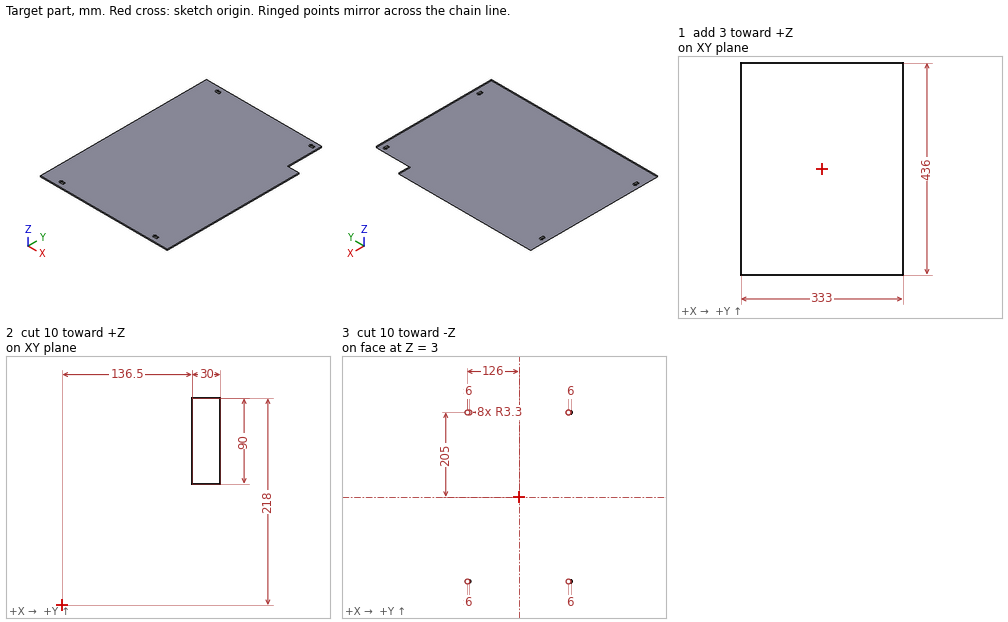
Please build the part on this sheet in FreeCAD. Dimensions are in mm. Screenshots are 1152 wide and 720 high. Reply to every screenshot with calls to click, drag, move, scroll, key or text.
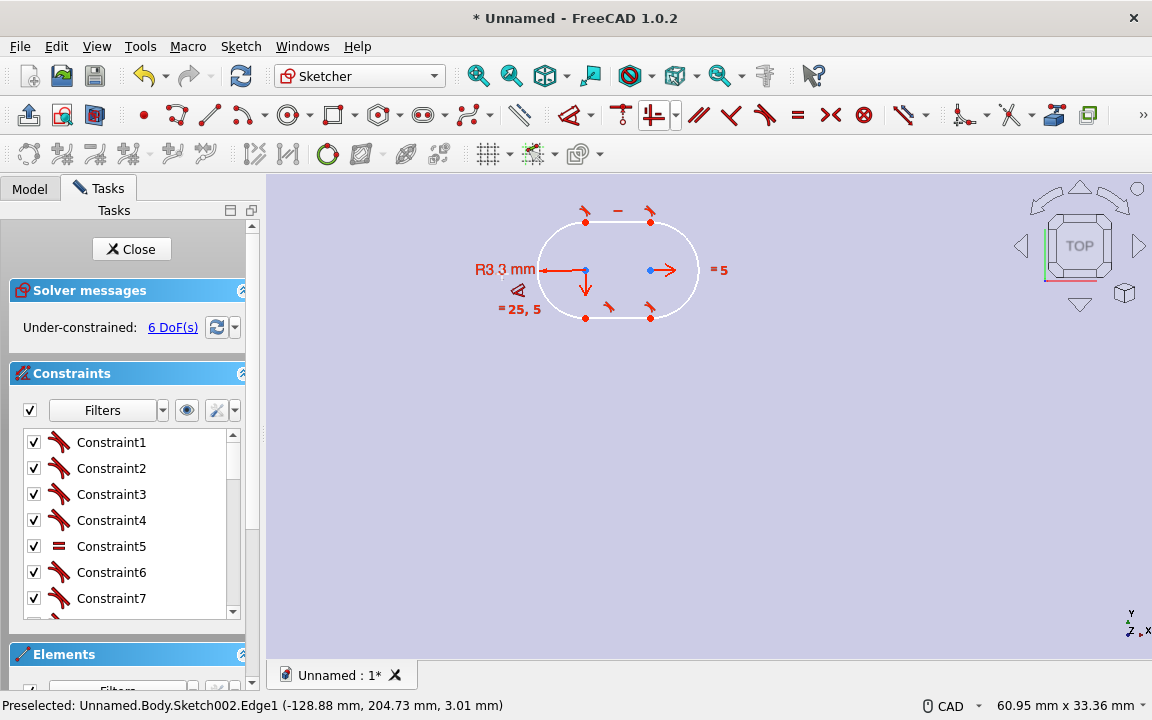
click(605, 222)
click(618, 256)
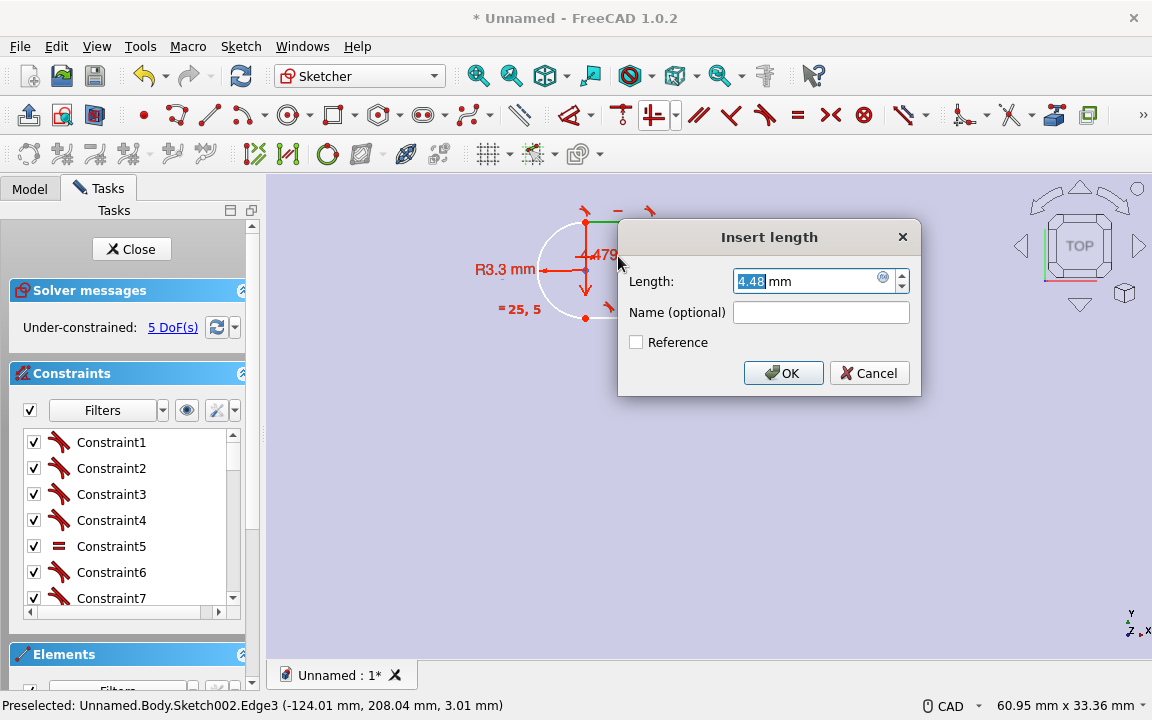
text(6)
key(Return)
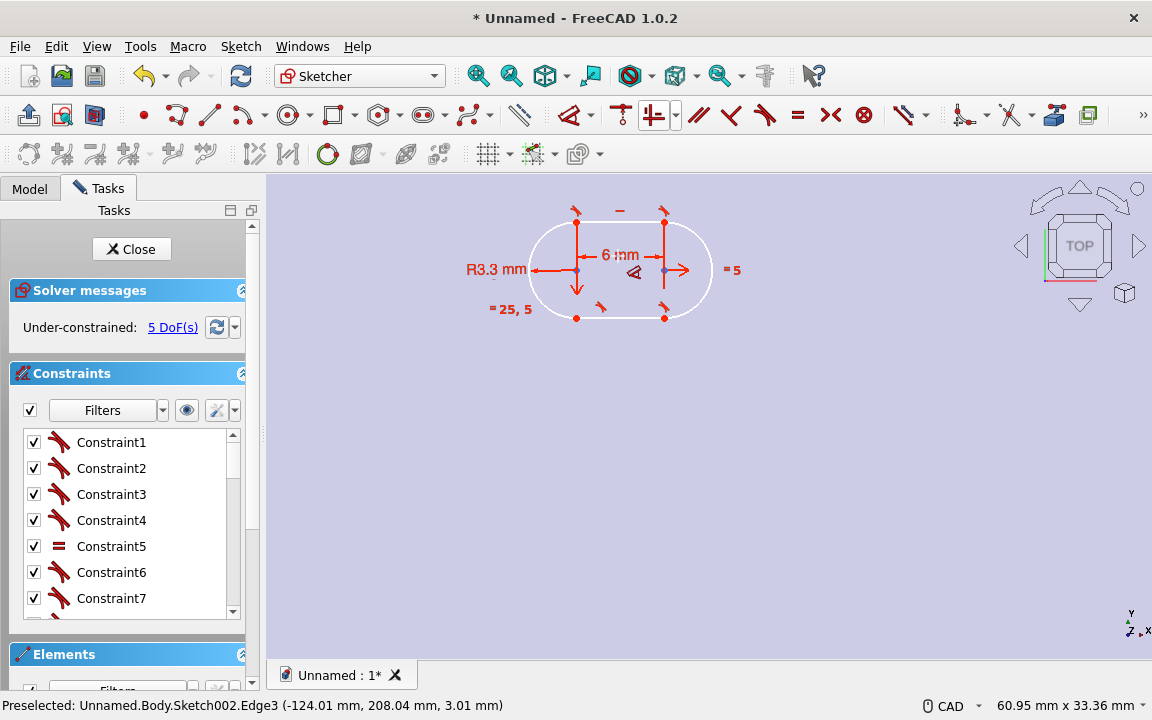
scroll(548, 268, down, 15)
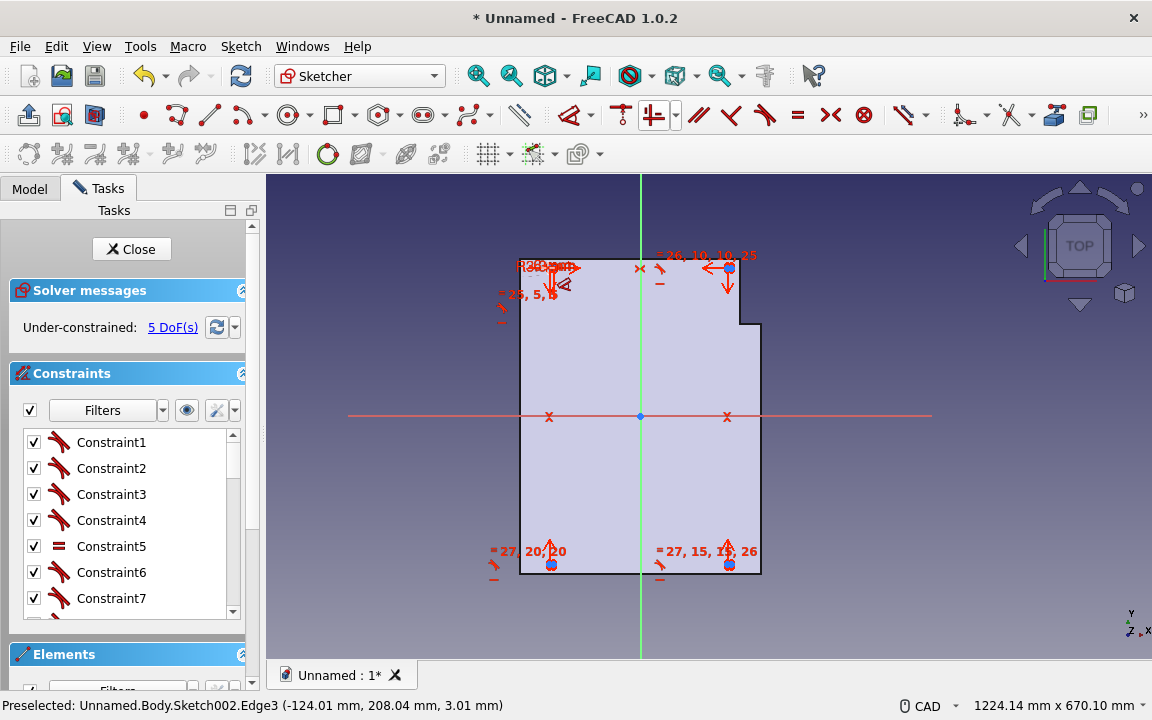
scroll(729, 266, up, 13)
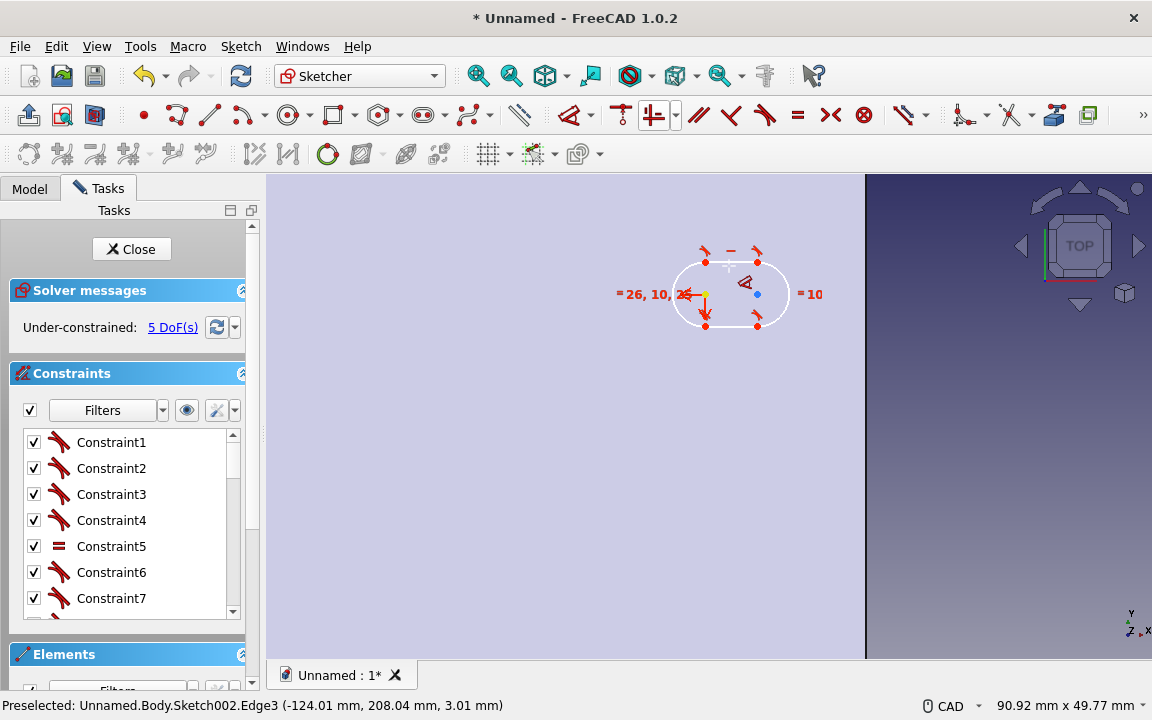
click(721, 262)
click(731, 228)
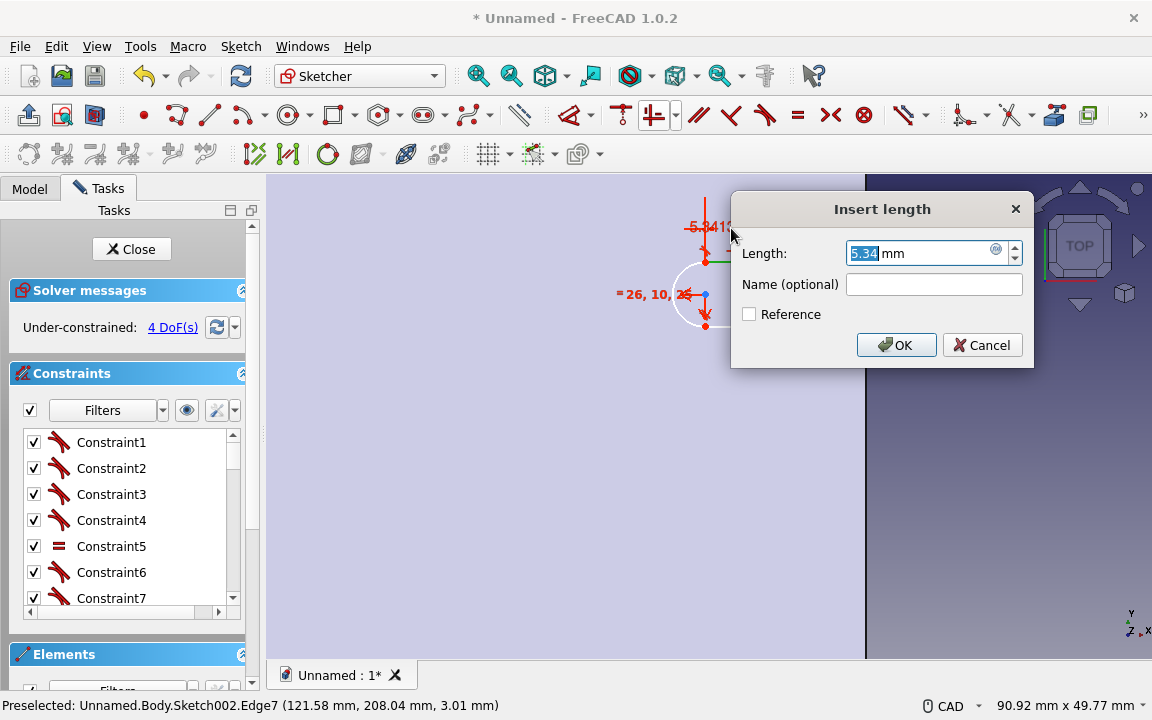
text(6)
key(Return)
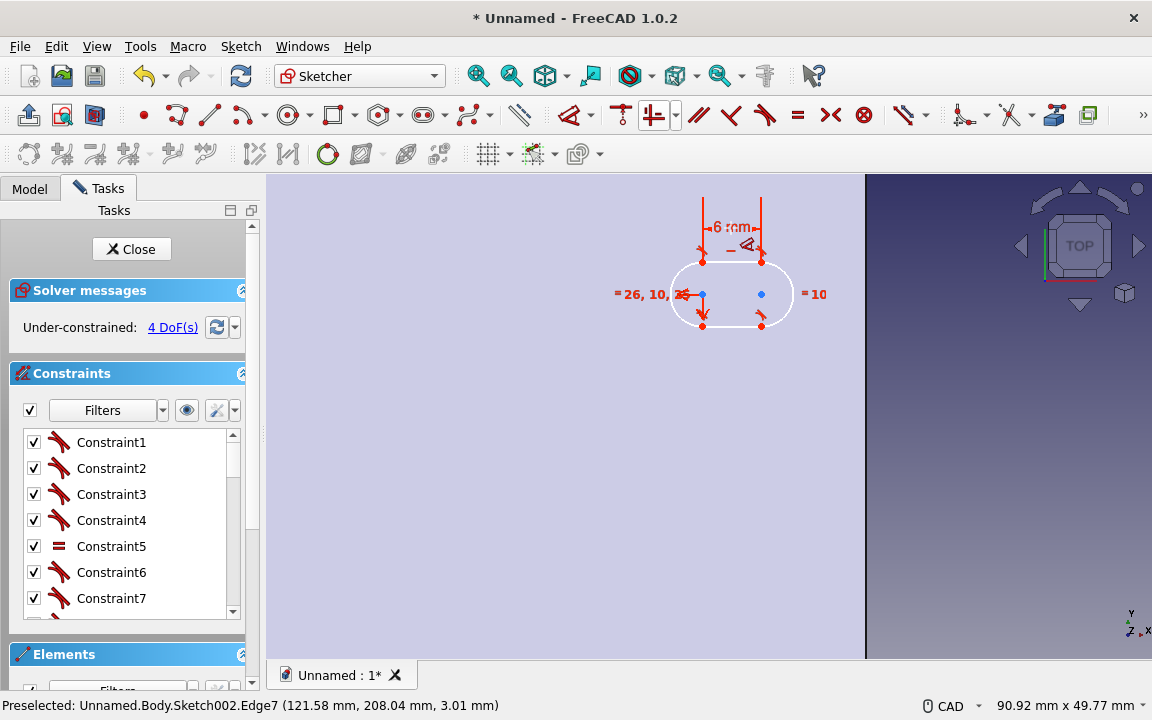
scroll(729, 266, down, 13)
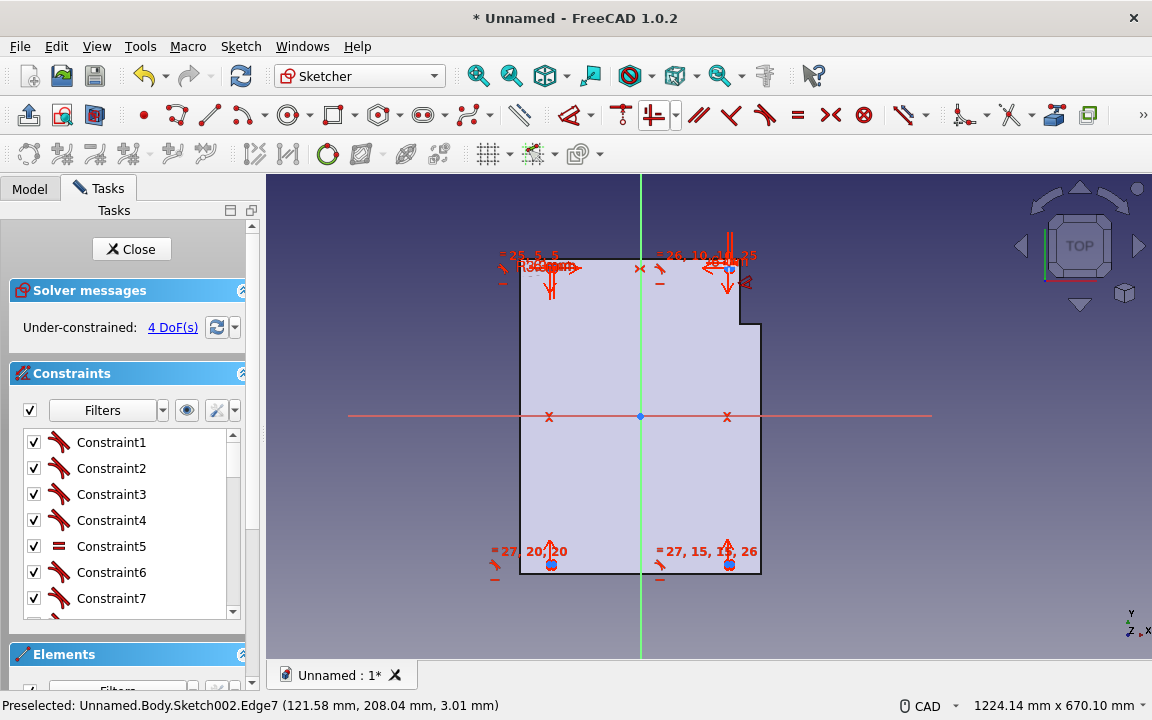
scroll(729, 562, up, 13)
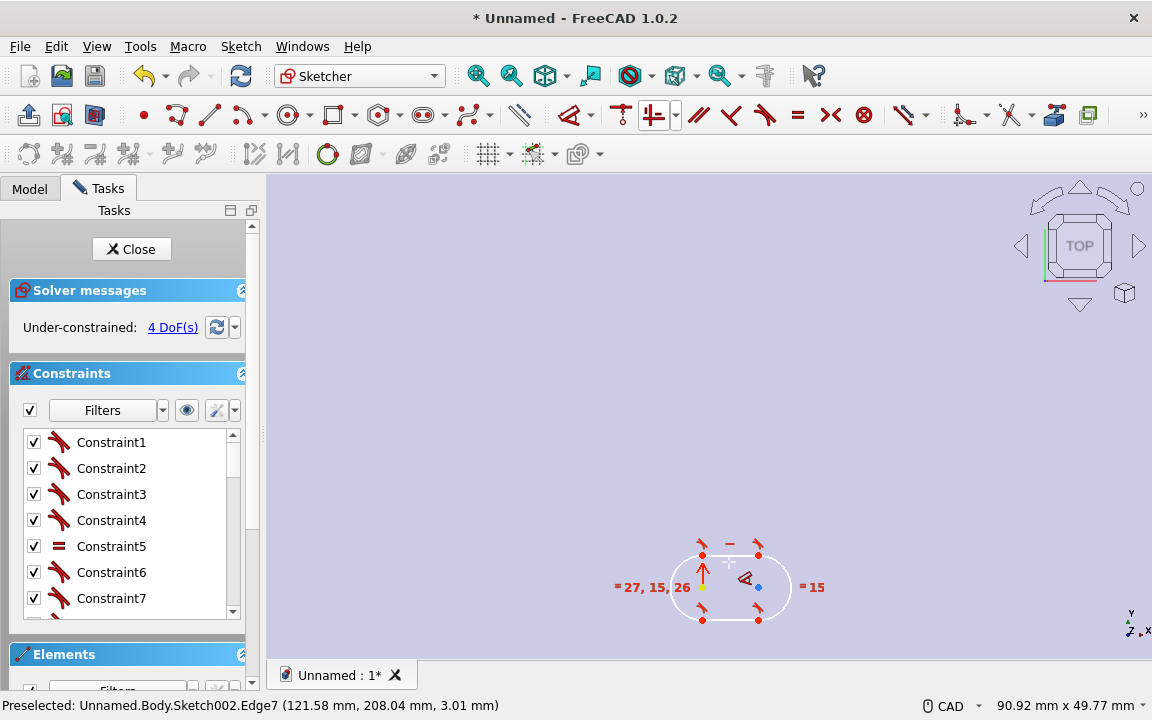
click(720, 556)
click(731, 590)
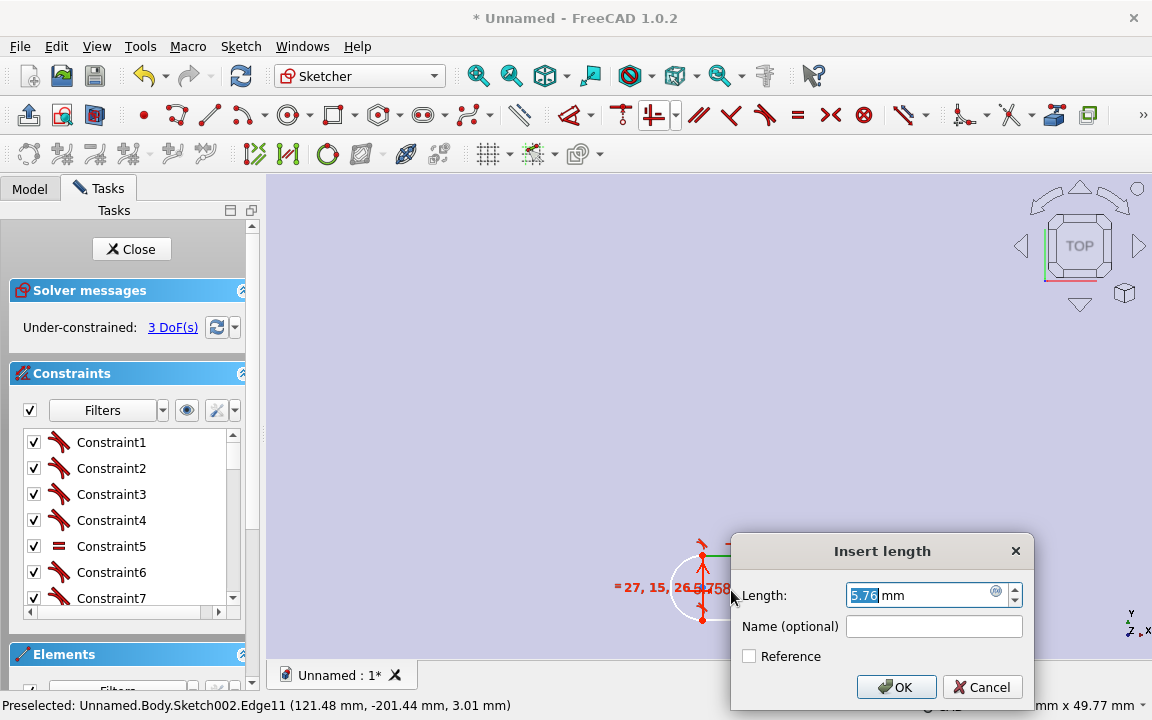
text(6)
key(Return)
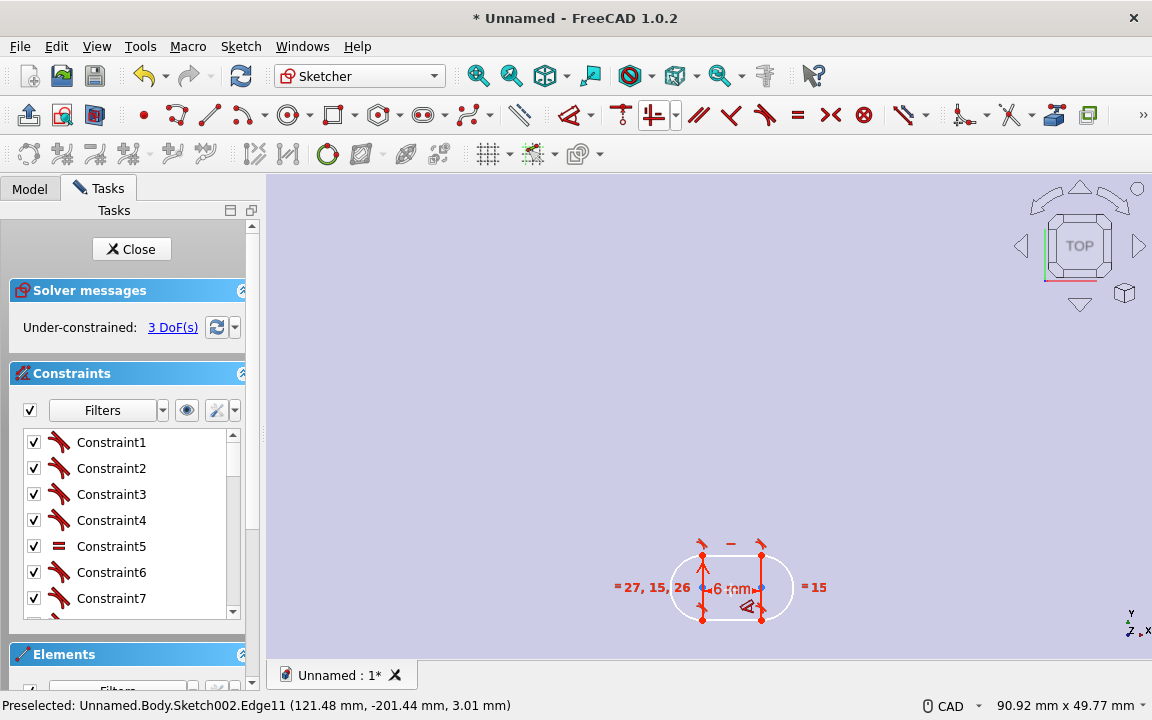
scroll(729, 563, down, 13)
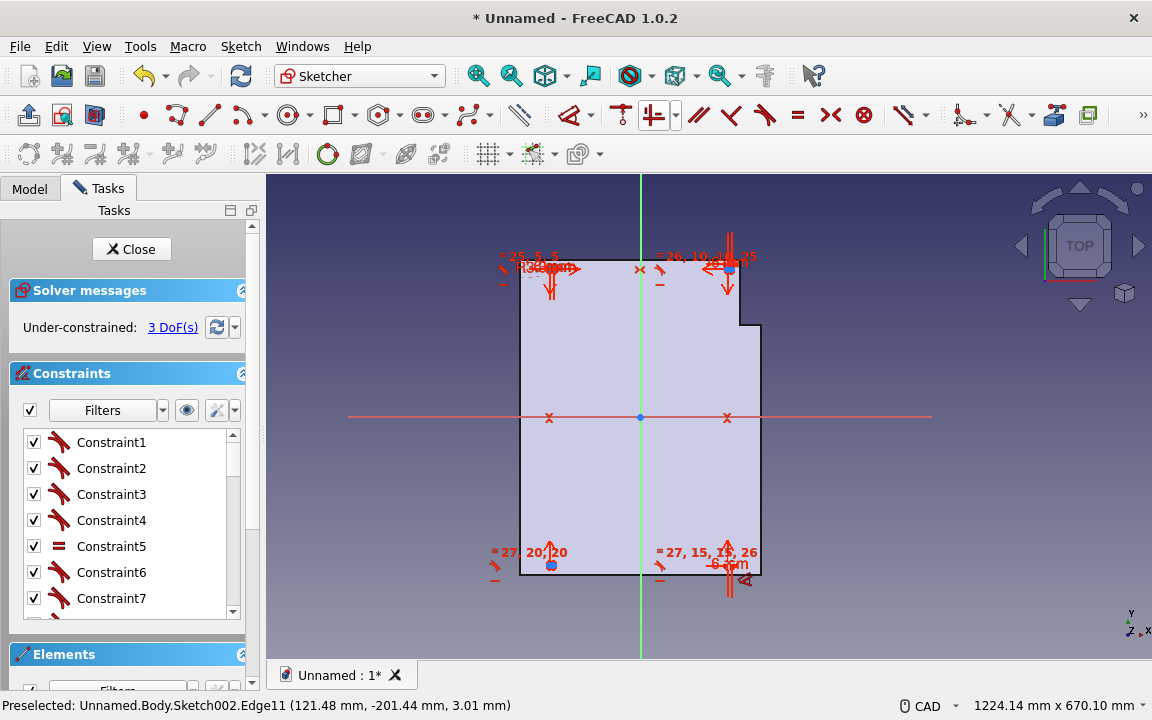
scroll(551, 563, up, 13)